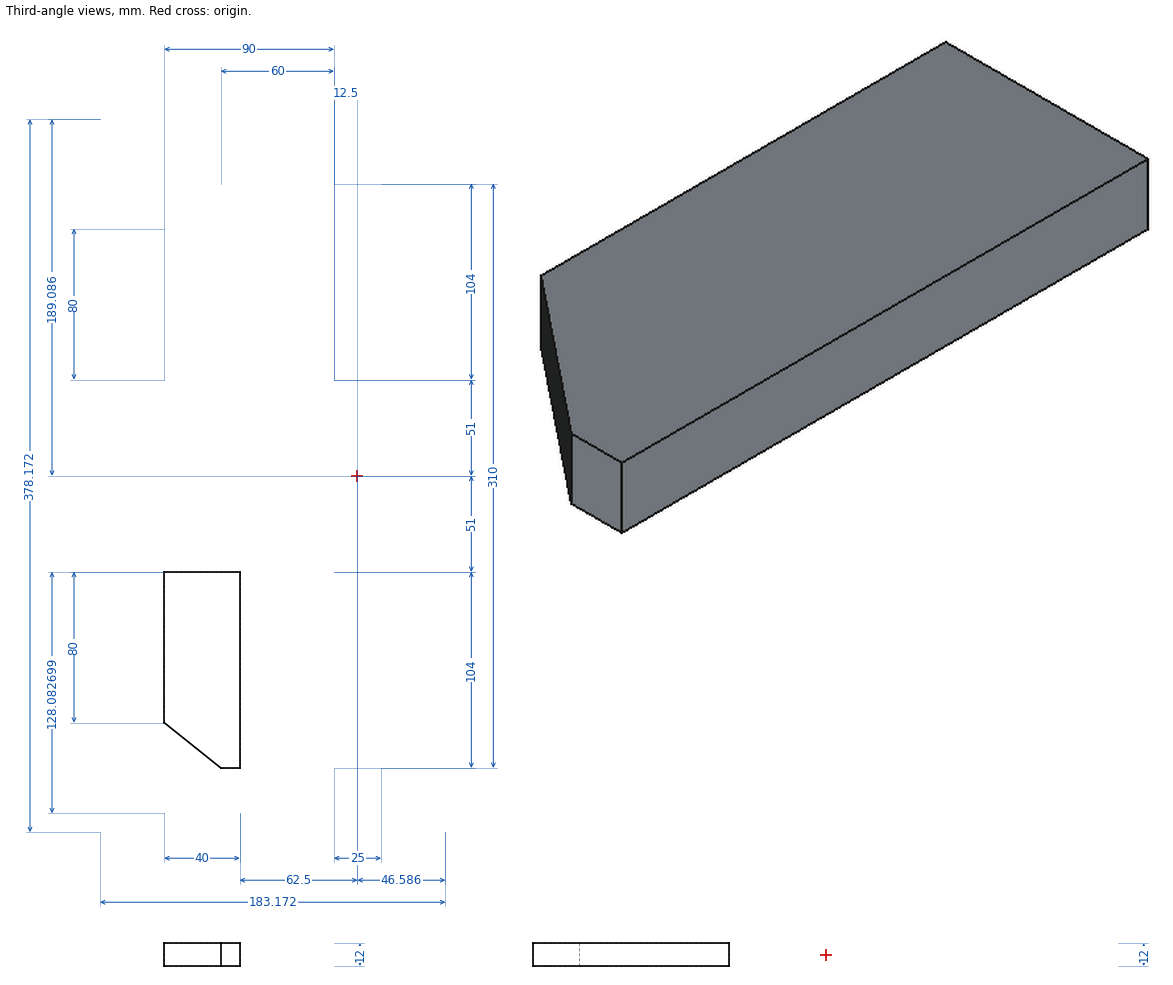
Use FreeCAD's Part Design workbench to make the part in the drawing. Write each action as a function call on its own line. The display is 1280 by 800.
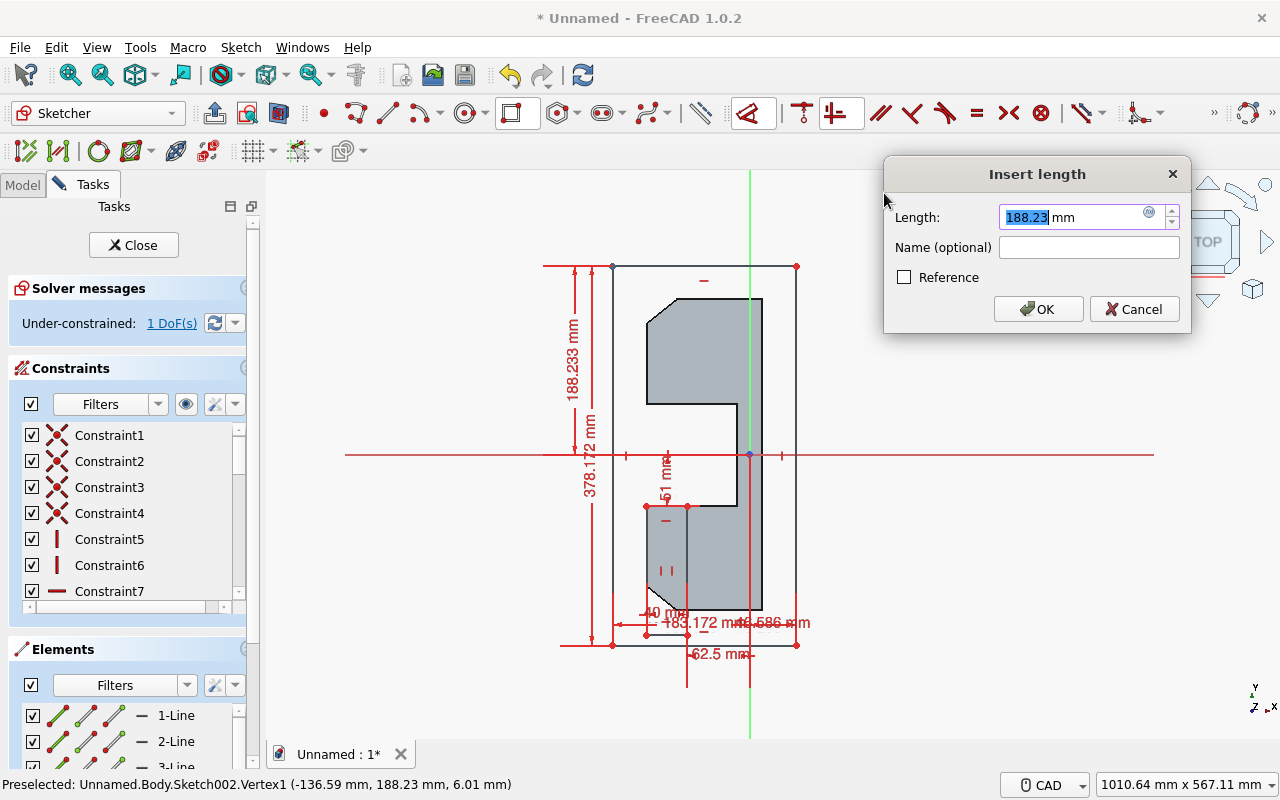
text(189.086)
key(Return)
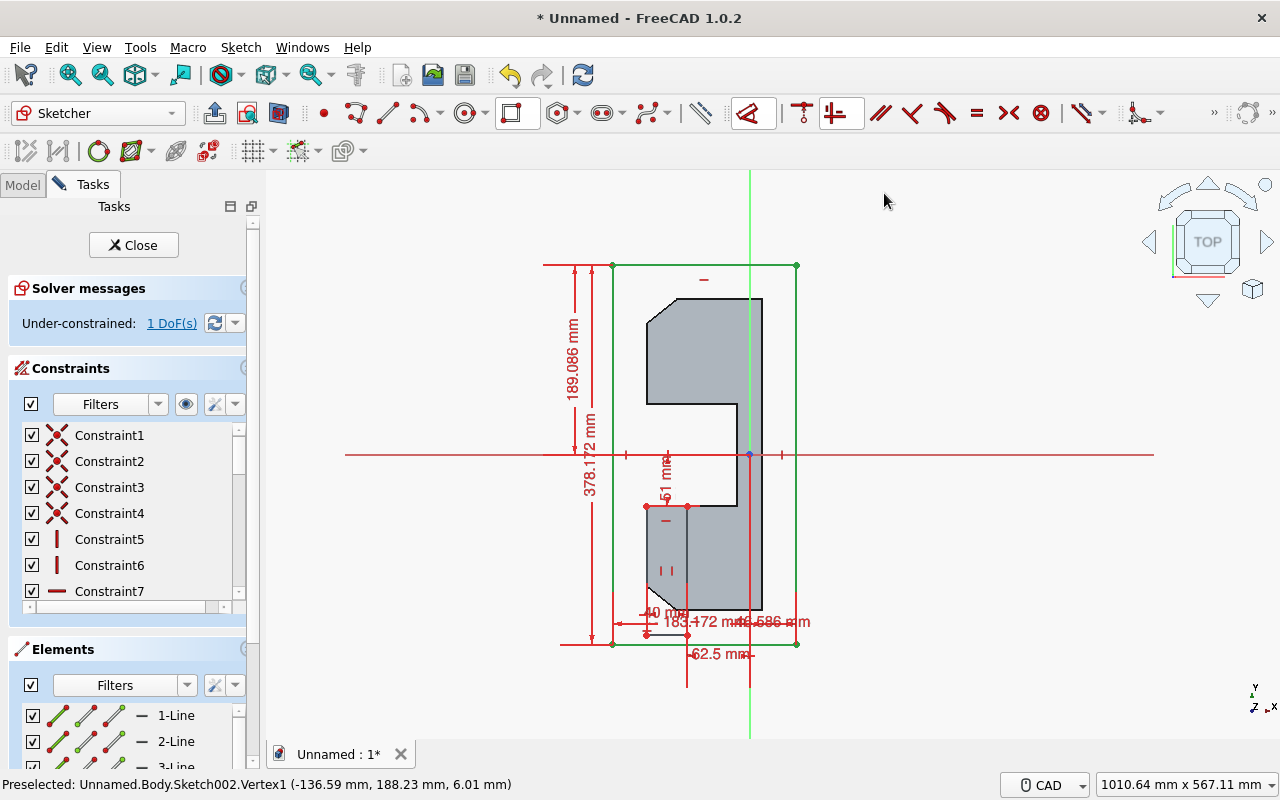
click(647, 545)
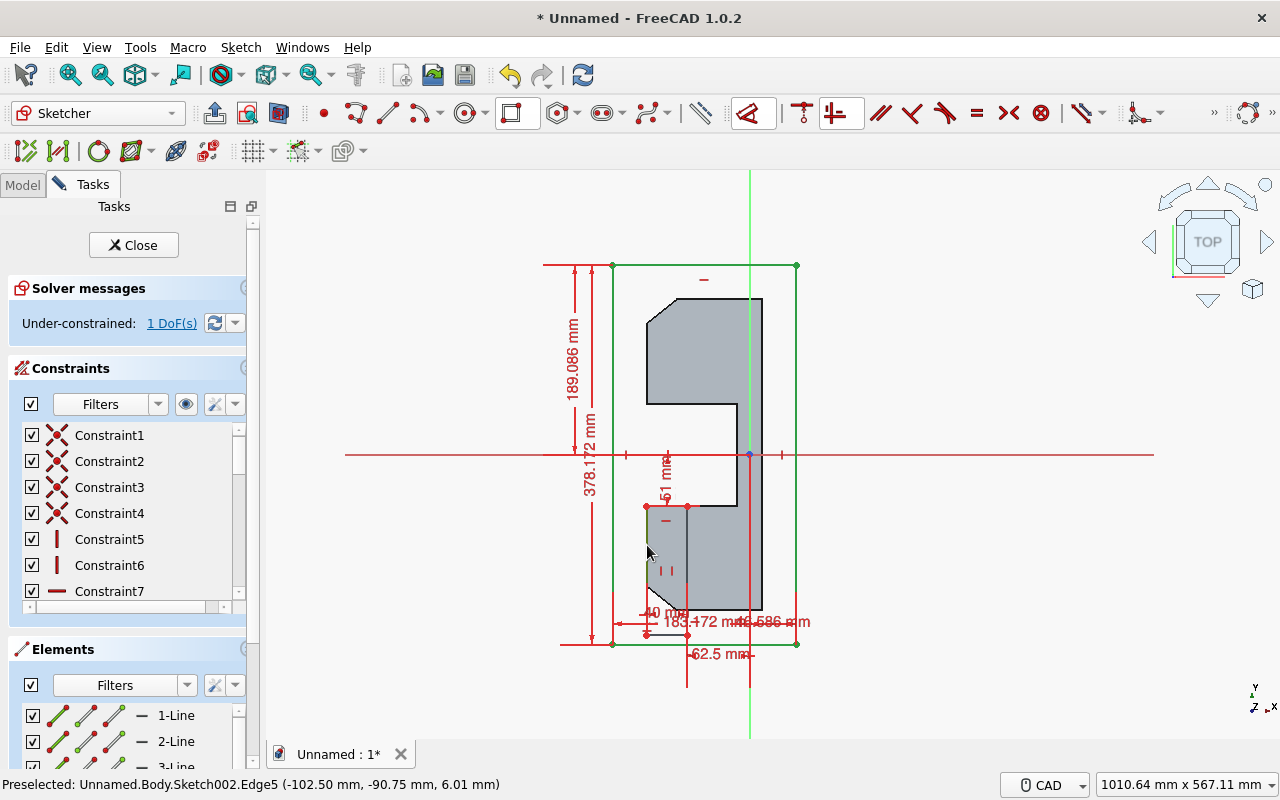
key(i)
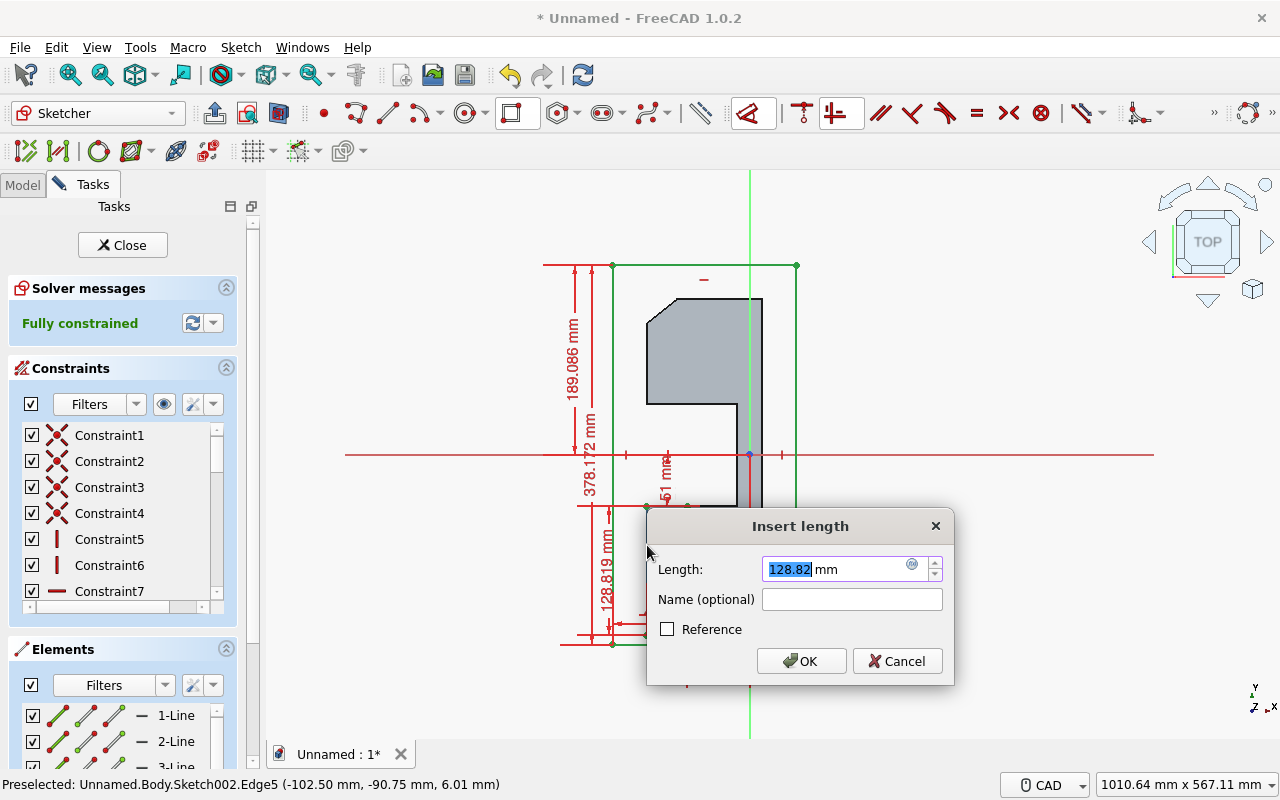
text(128.082699)
key(Return)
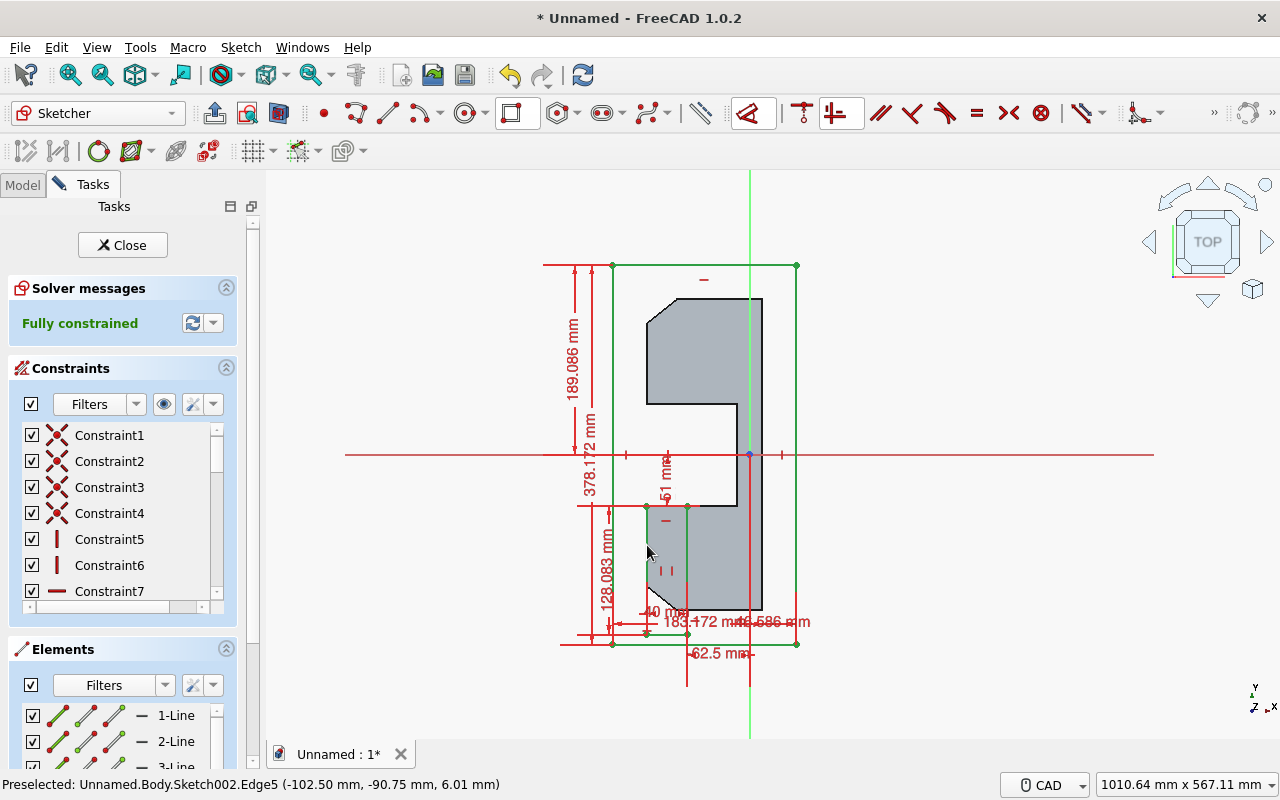
click(123, 245)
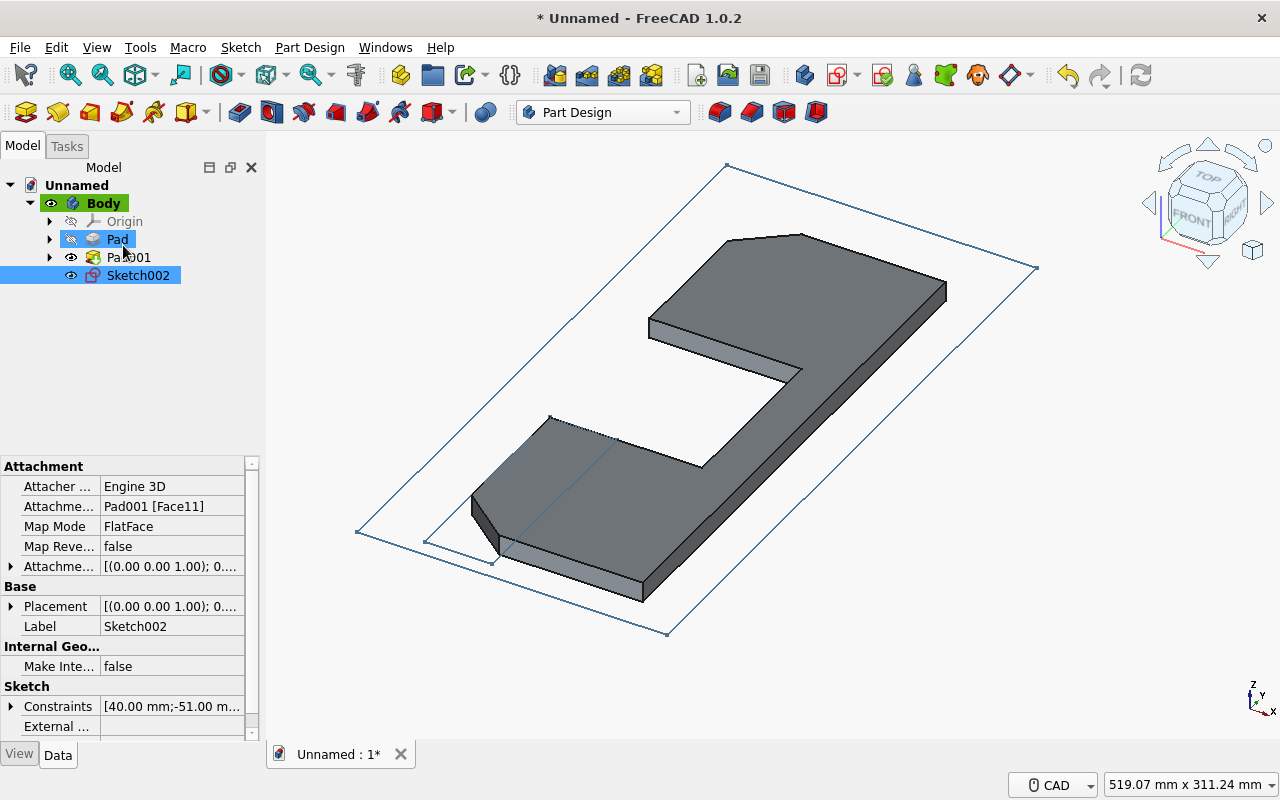
click(240, 112)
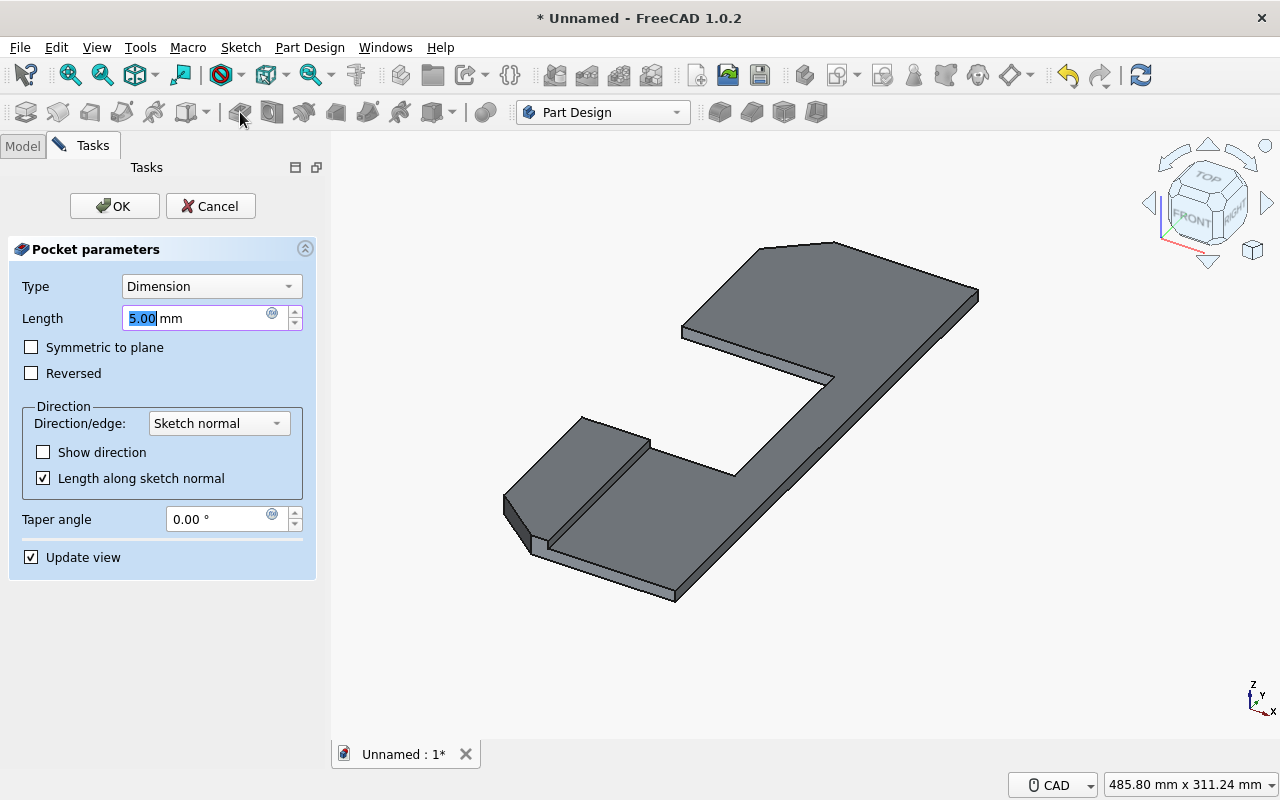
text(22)
key(Tab)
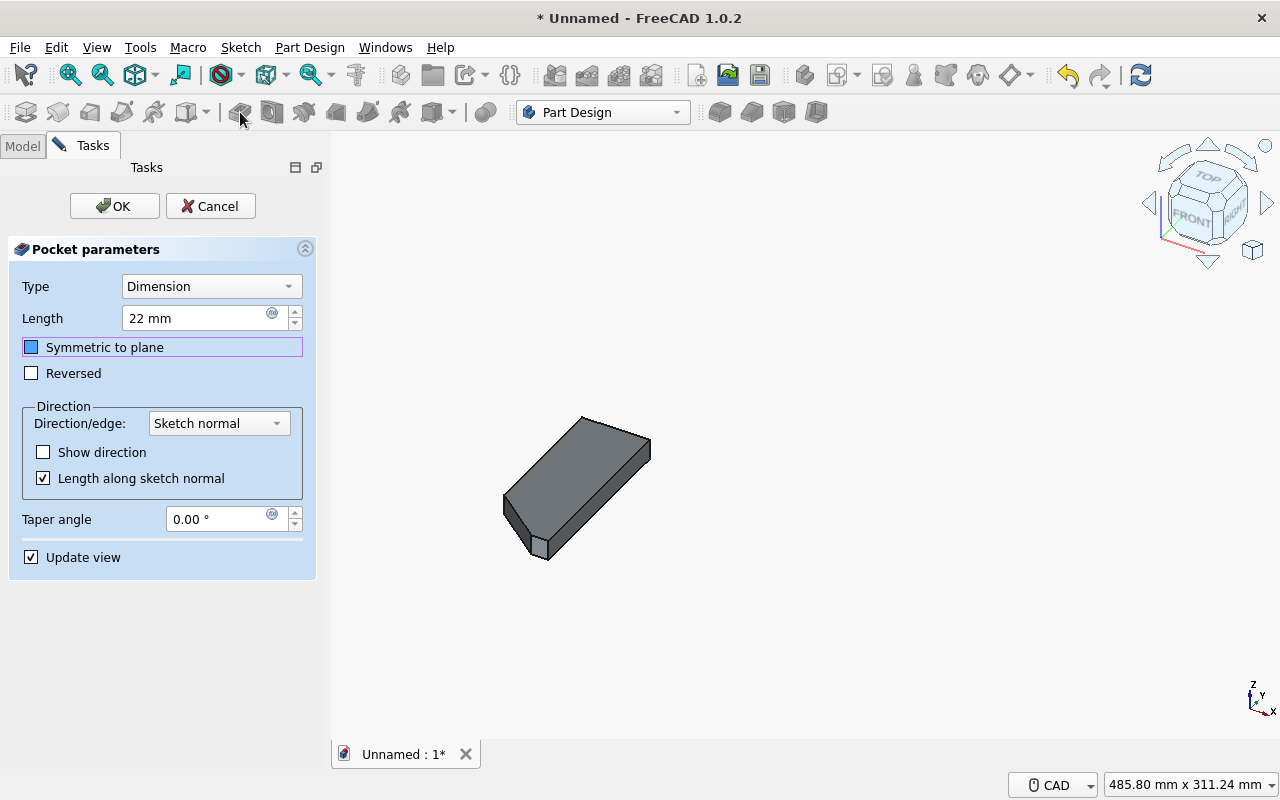
click(115, 206)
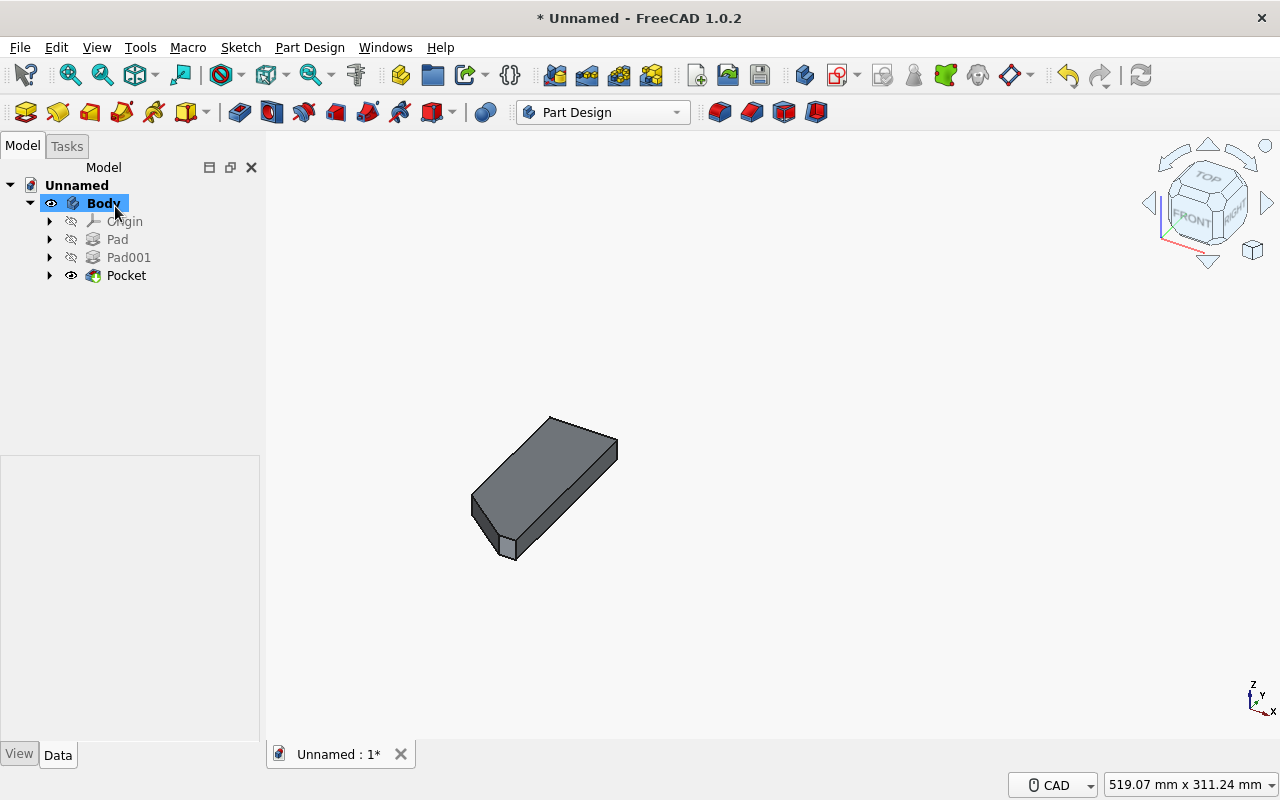
key(0)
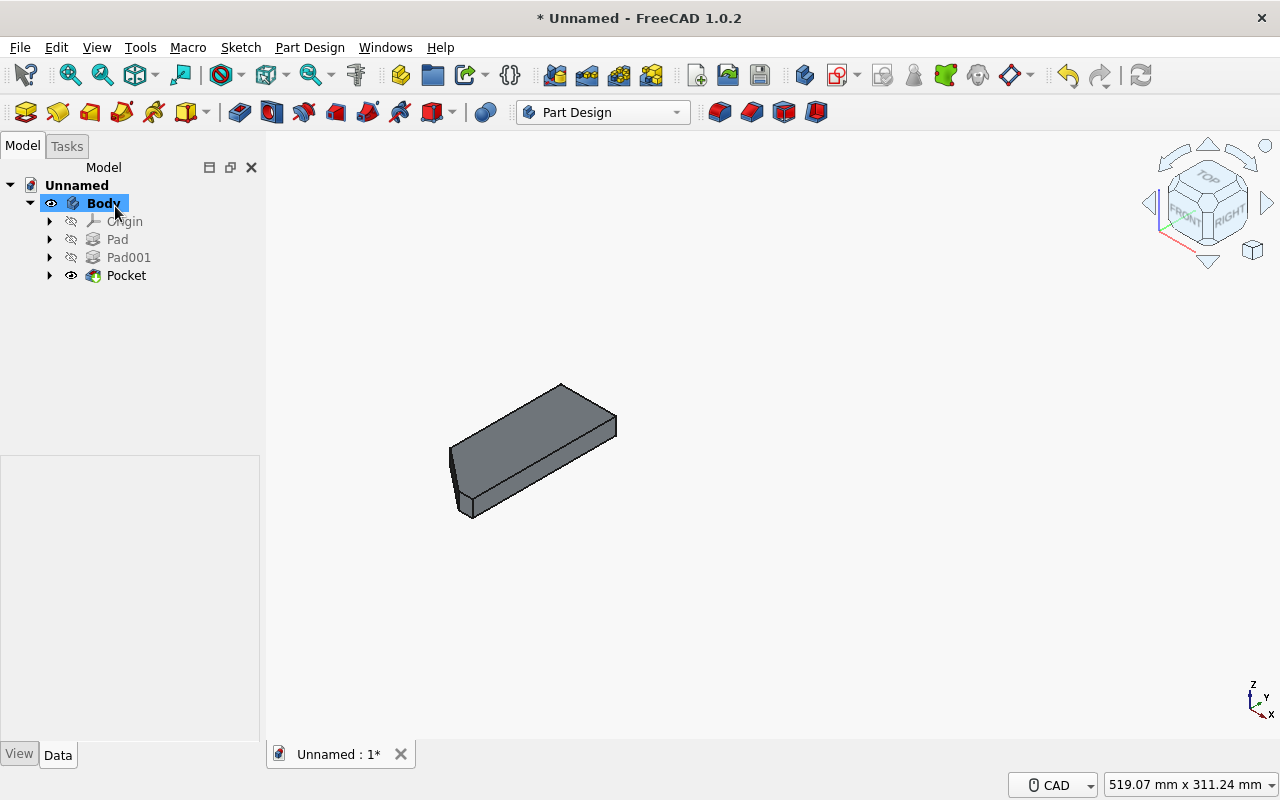
click(72, 76)